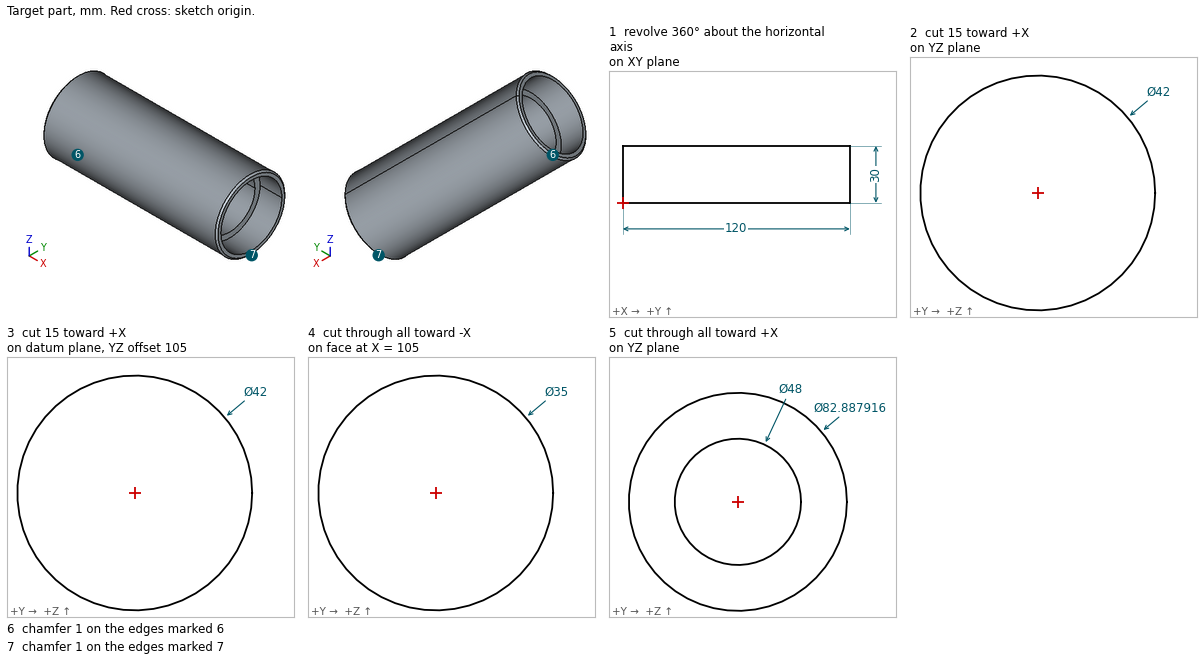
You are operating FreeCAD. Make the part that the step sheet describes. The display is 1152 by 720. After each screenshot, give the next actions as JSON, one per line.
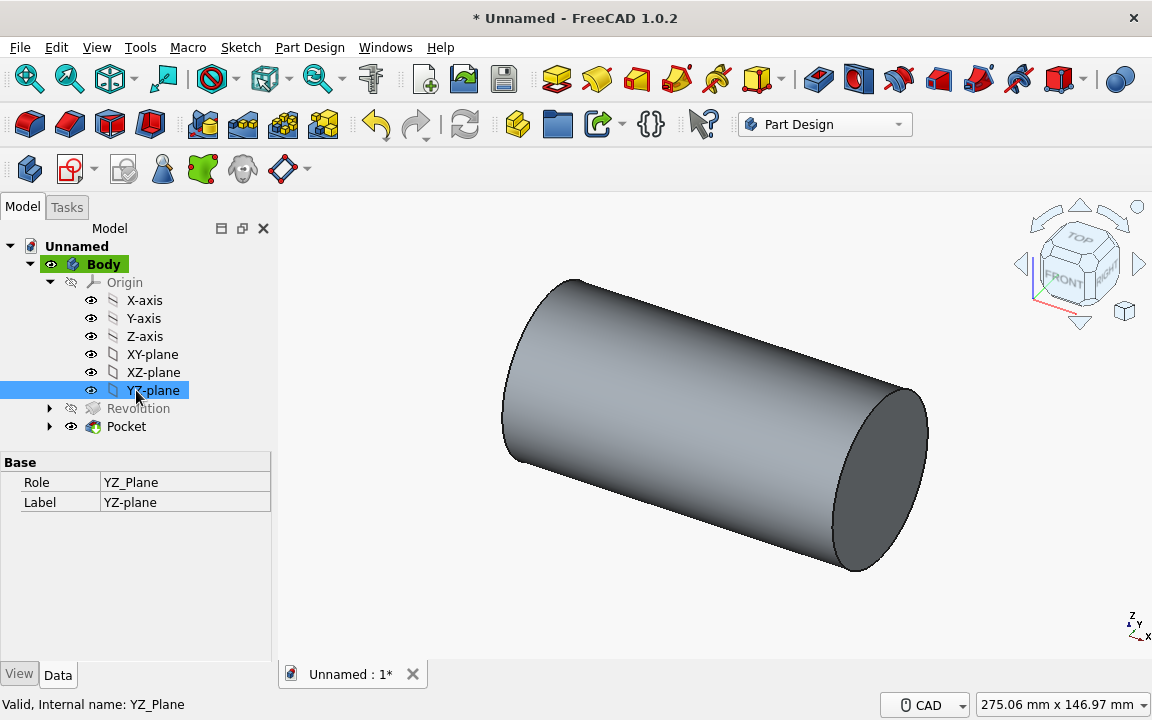
{"action": "left_click", "coordinate": [284, 170]}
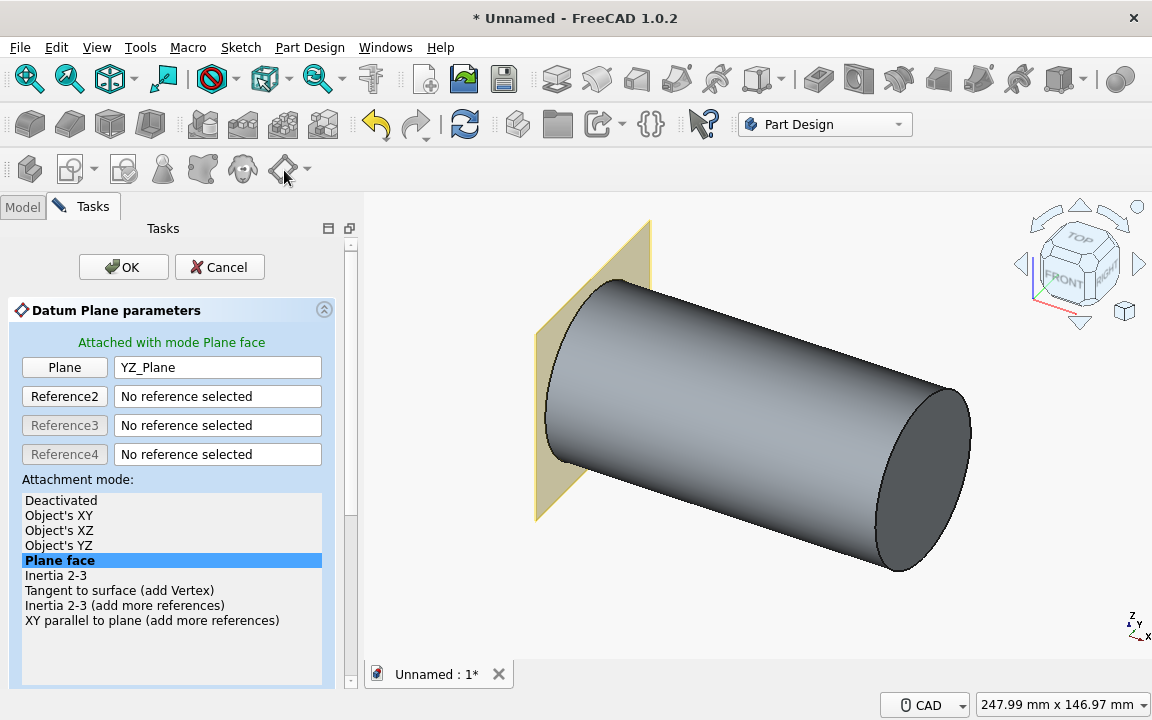
{"action": "scroll", "coordinate": [351, 463], "scroll_direction": "down", "scroll_amount": 3}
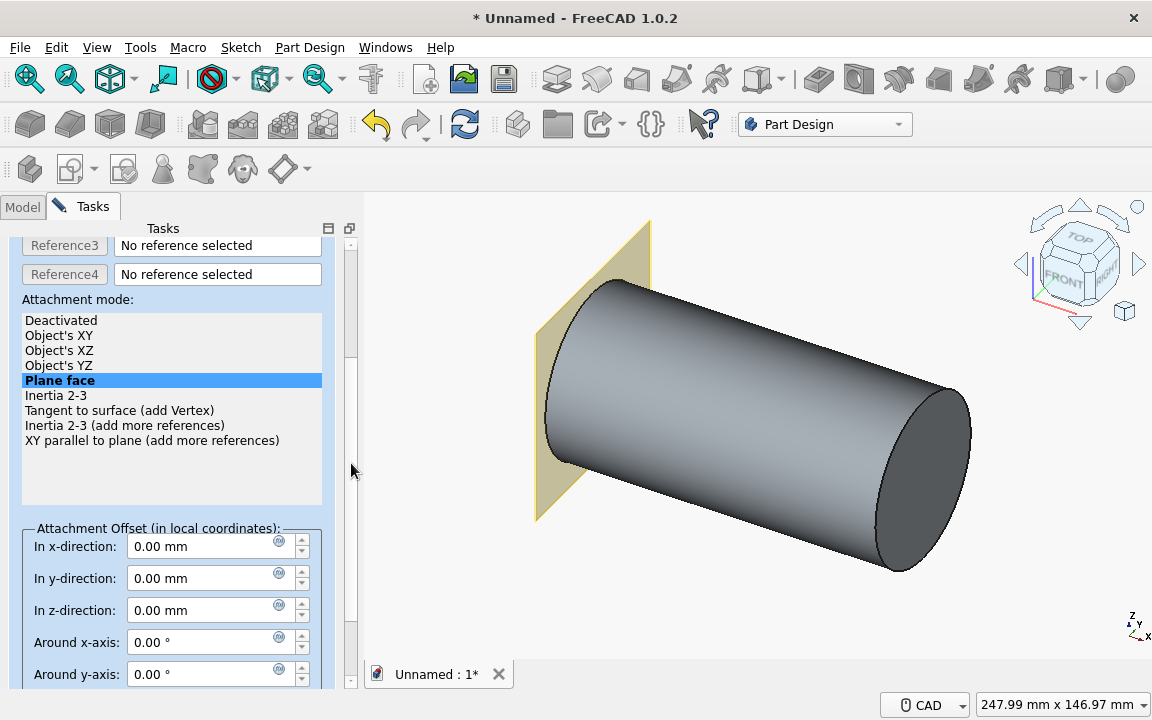
{"action": "triple_click", "coordinate": [210, 610]}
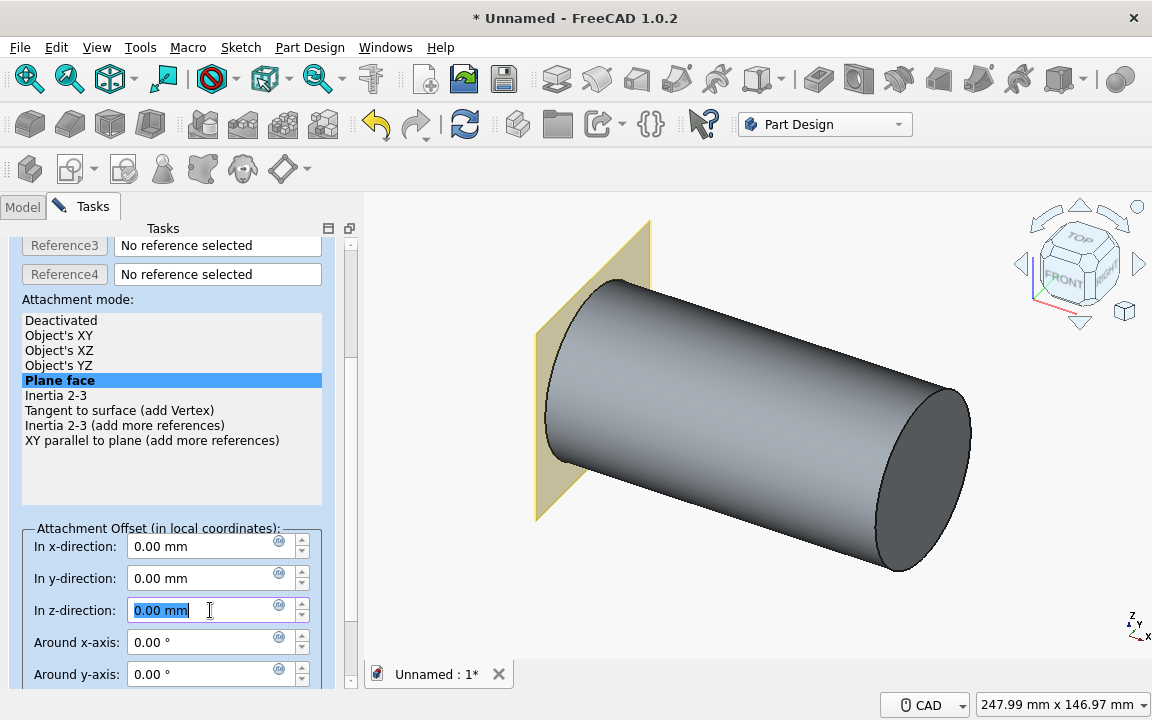
{"action": "type", "text": "105"}
{"action": "key", "text": "Tab"}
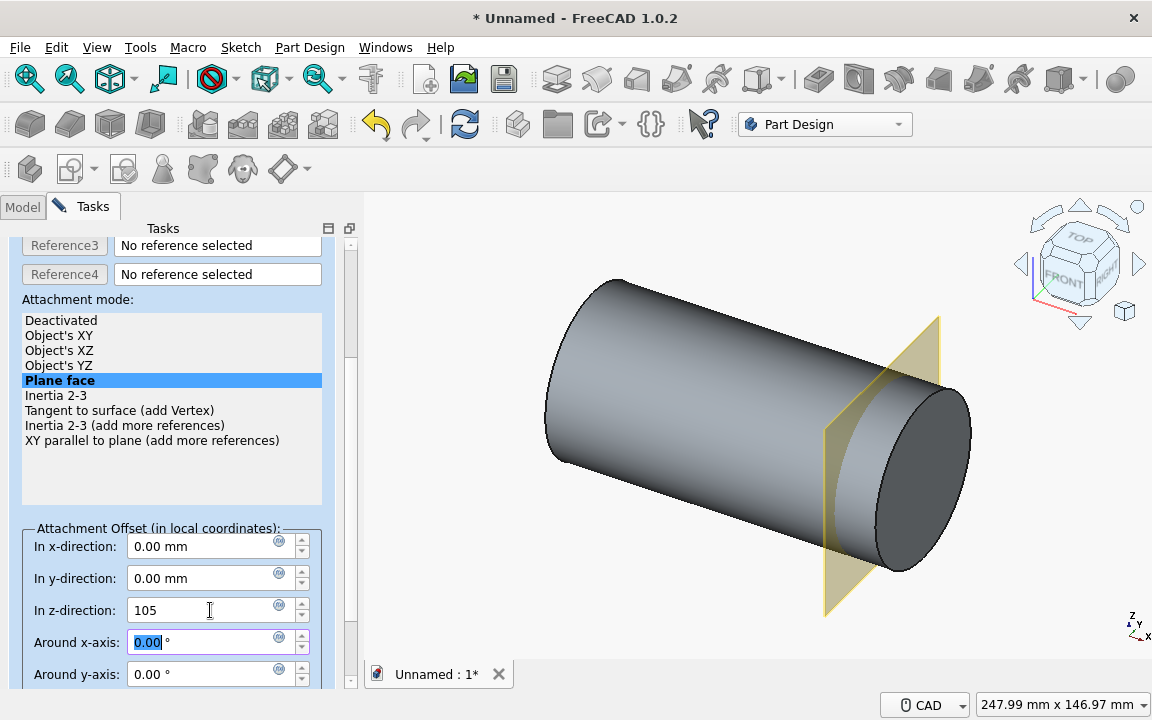
{"action": "scroll", "coordinate": [351, 463], "scroll_direction": "up", "scroll_amount": 4}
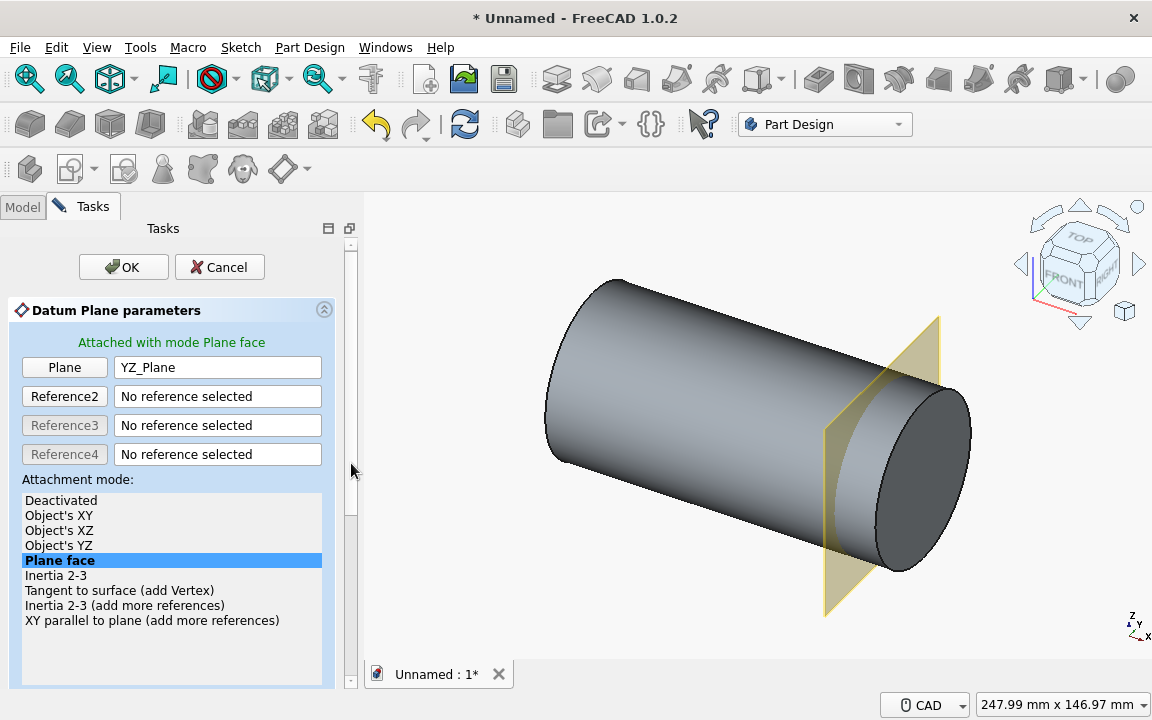
{"action": "left_click", "coordinate": [124, 267]}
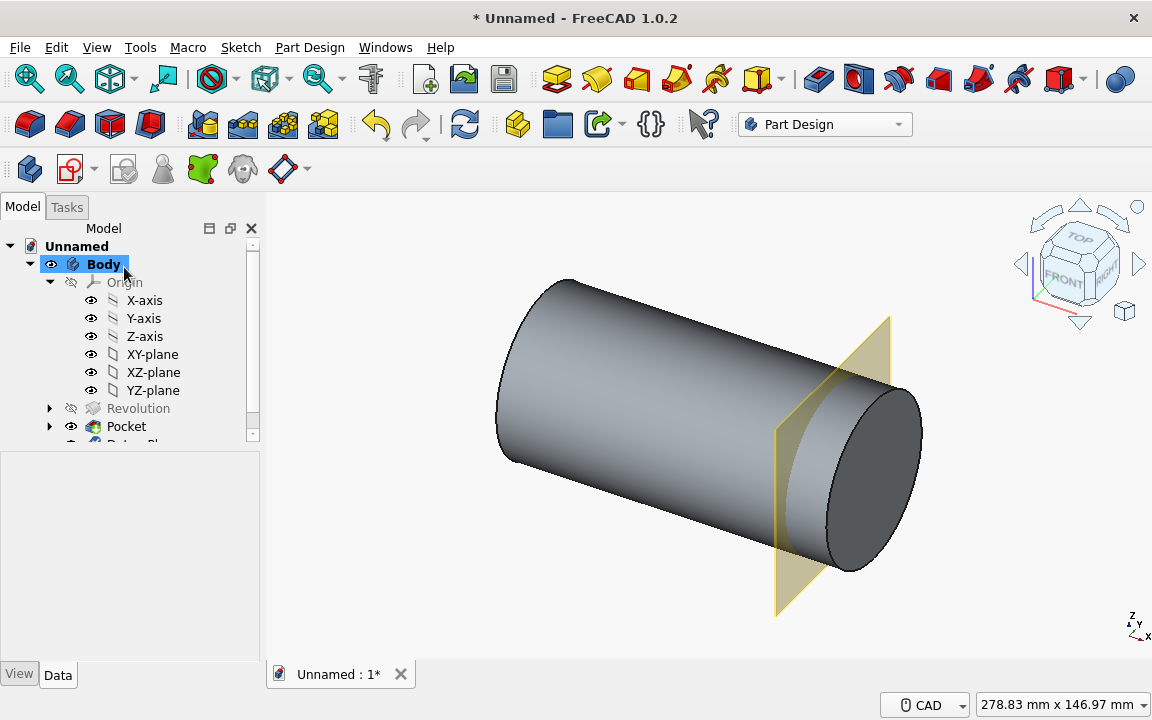
{"action": "scroll", "coordinate": [100, 332], "scroll_direction": "down", "scroll_amount": 3}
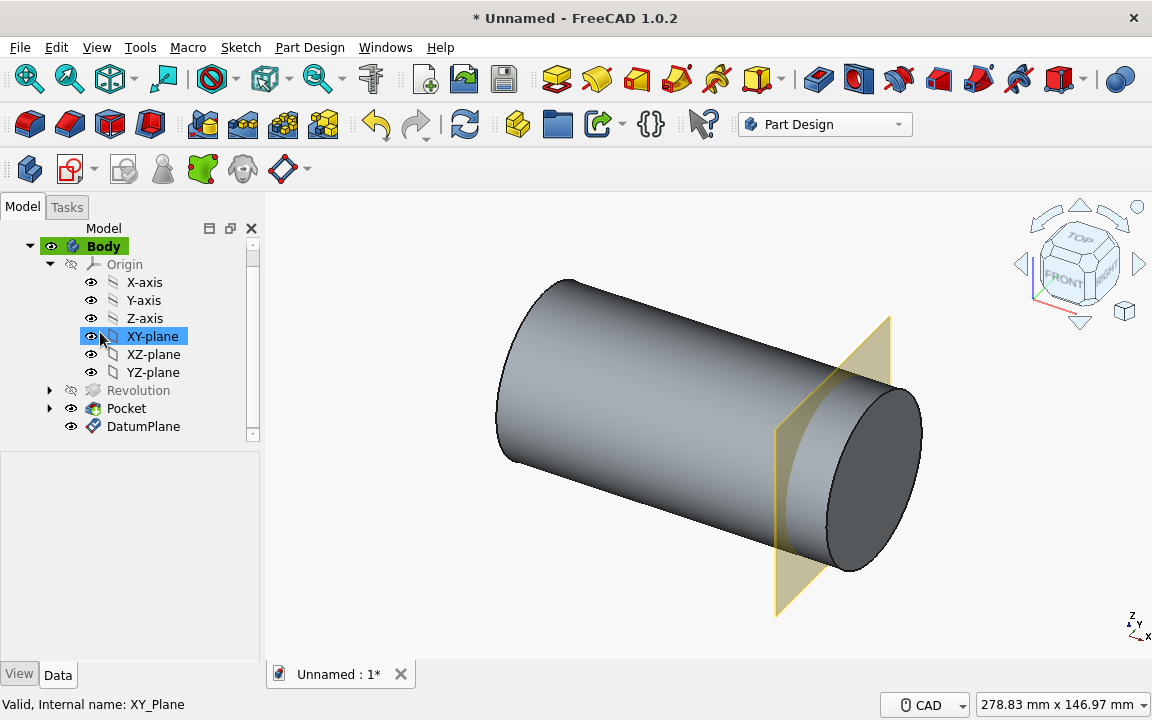
{"action": "left_click", "coordinate": [116, 426]}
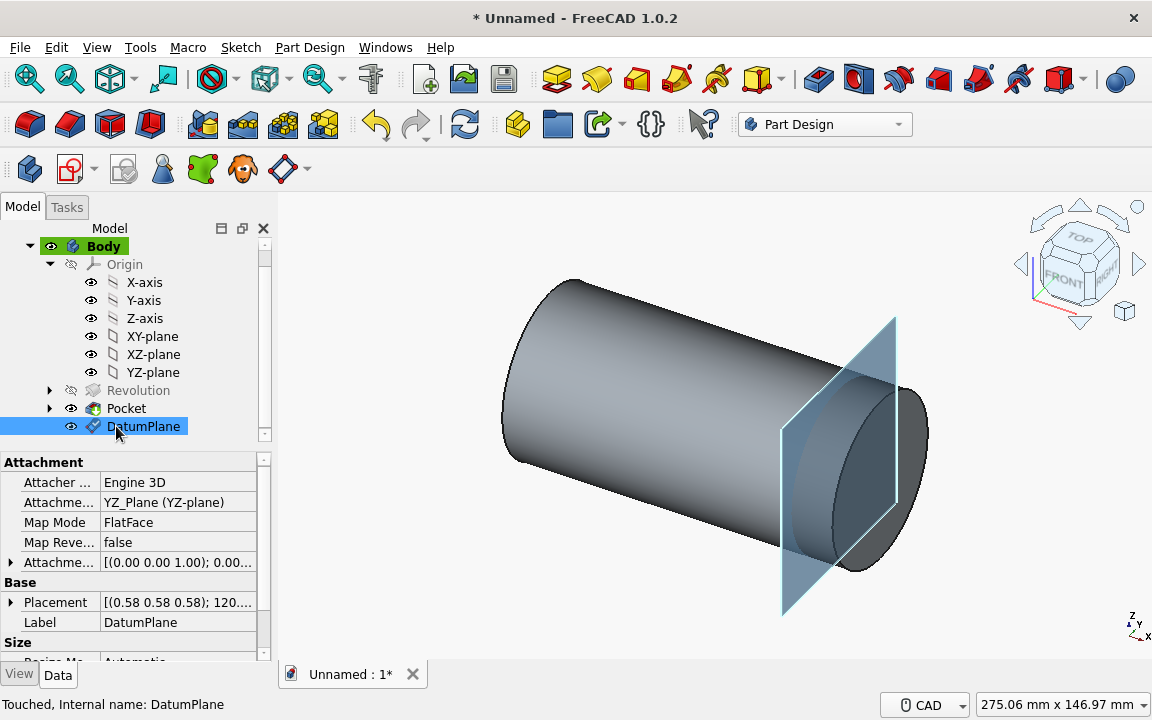
{"action": "left_click", "coordinate": [70, 170]}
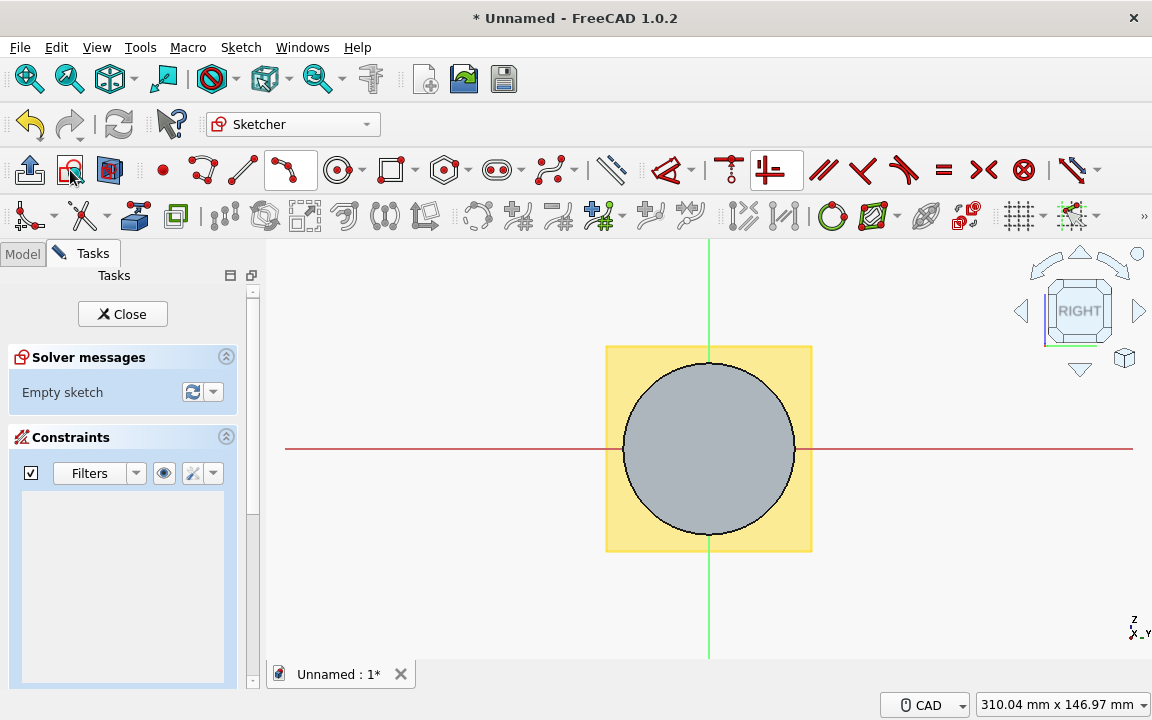
{"action": "key", "text": "q s"}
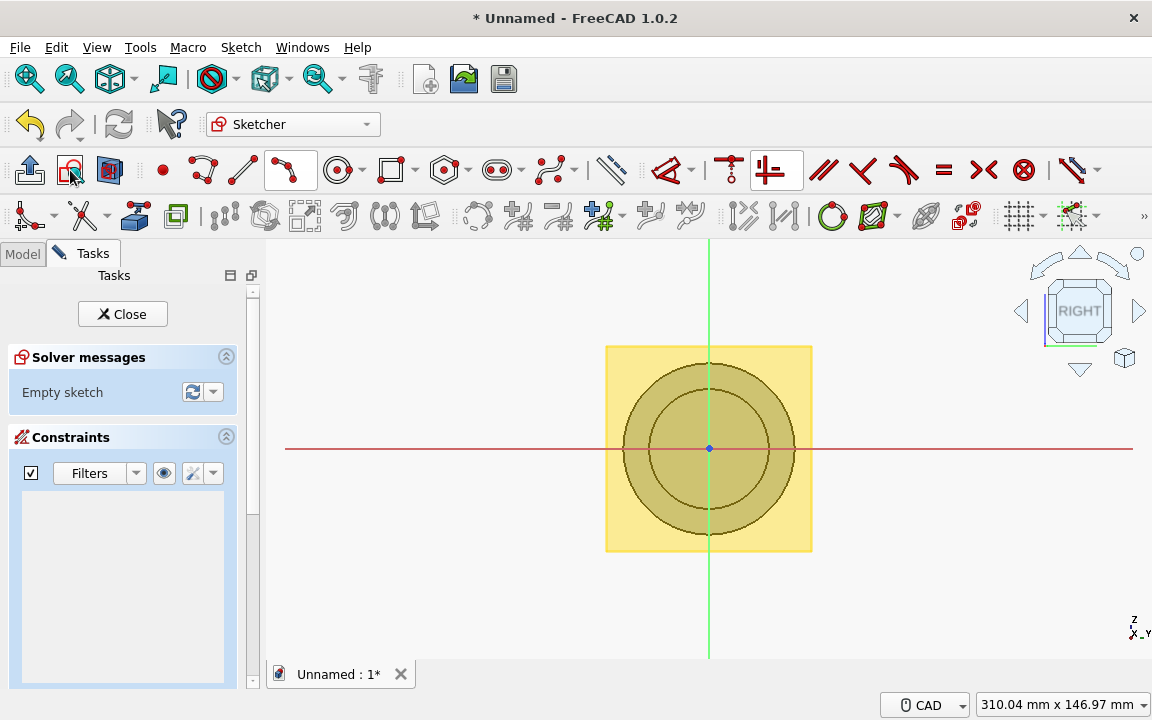
{"action": "scroll", "coordinate": [765, 449], "scroll_direction": "up", "scroll_amount": 4}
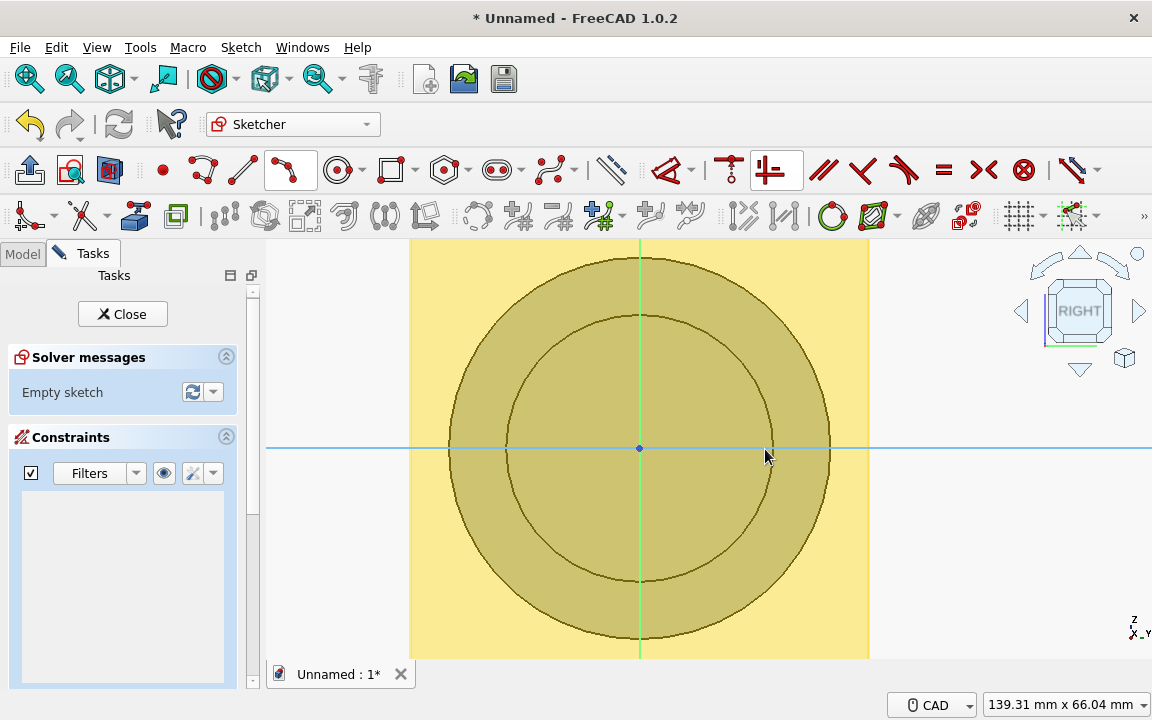
{"action": "key", "text": "g c"}